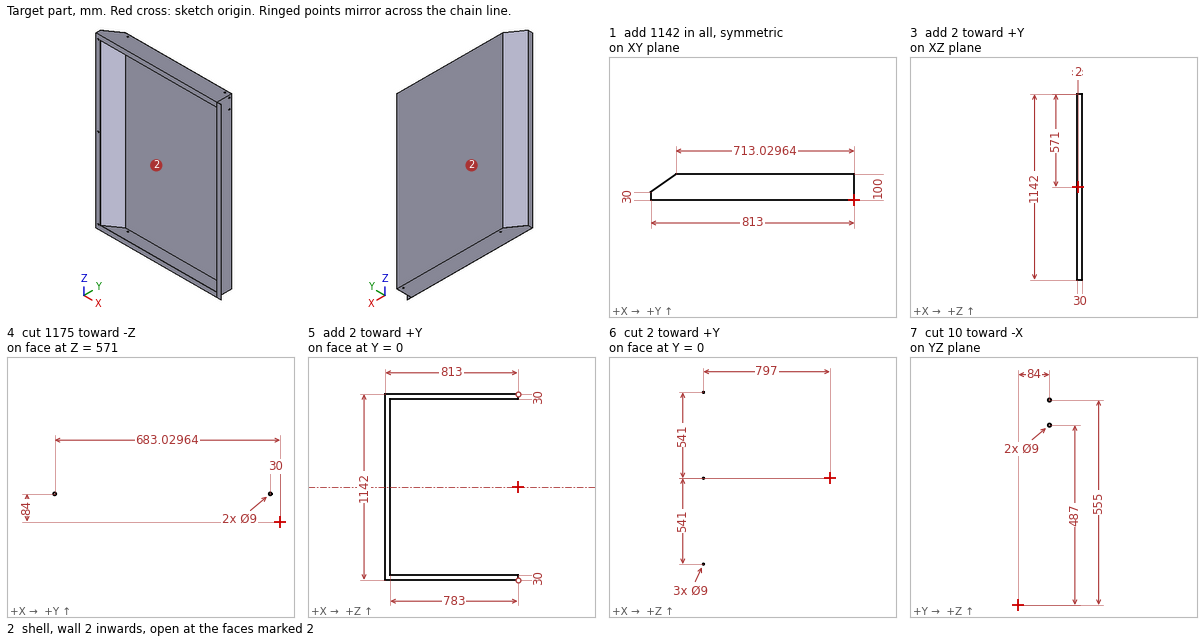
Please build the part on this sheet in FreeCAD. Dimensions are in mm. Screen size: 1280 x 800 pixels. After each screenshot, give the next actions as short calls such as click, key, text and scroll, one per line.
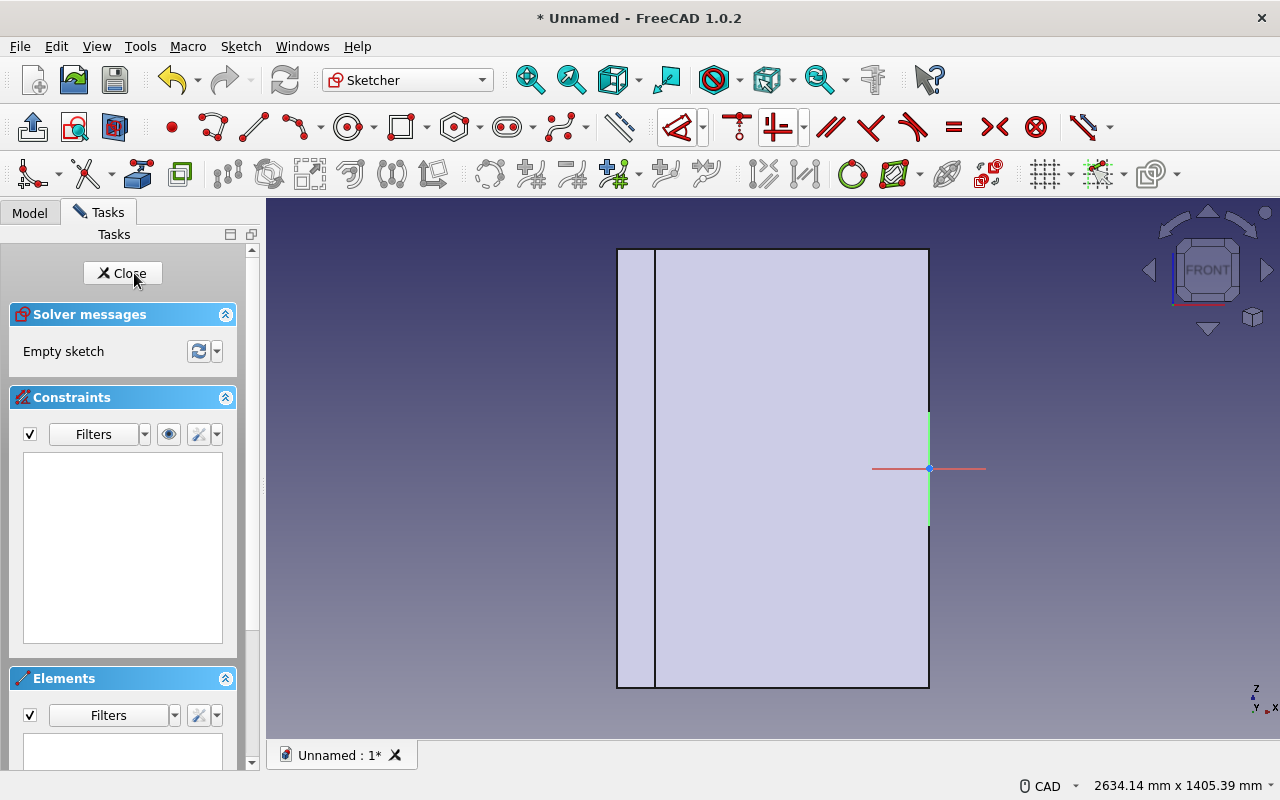
scroll(294, 468, down, 1)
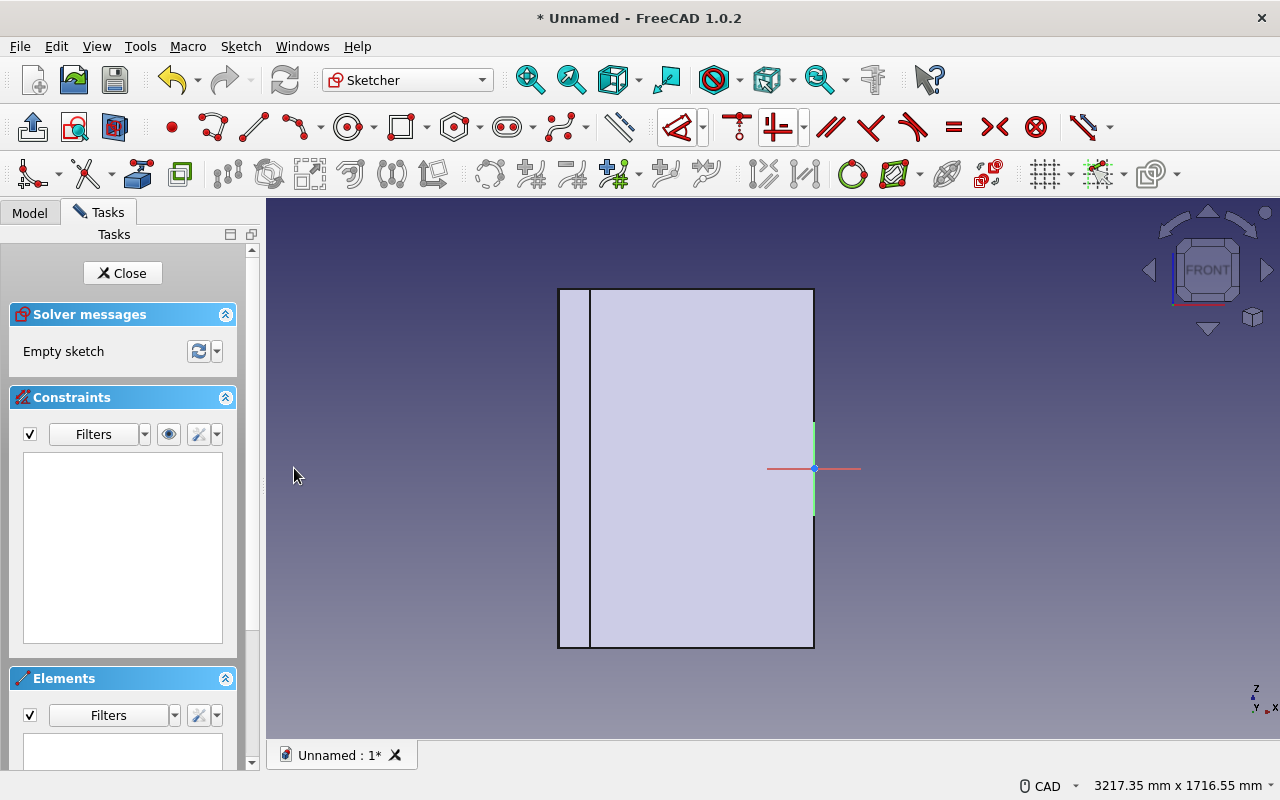
click(400, 128)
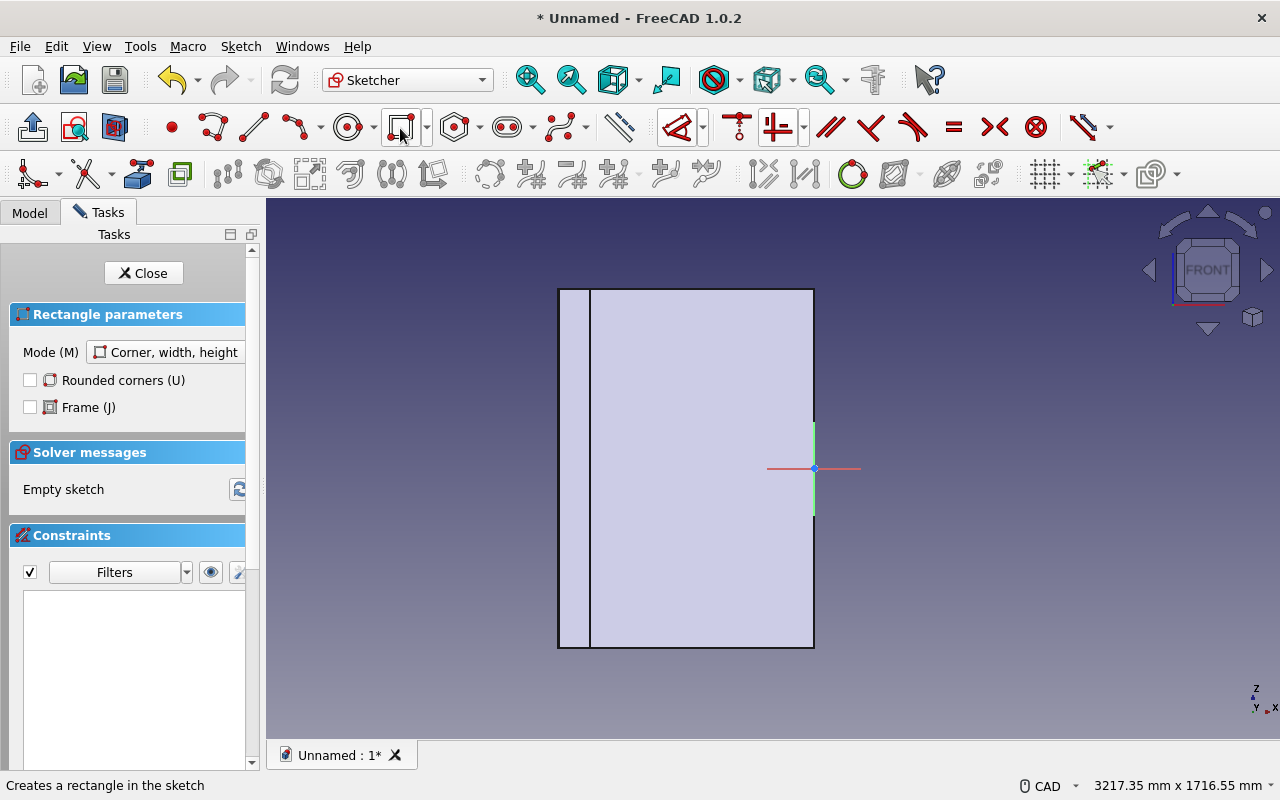
scroll(814, 289, up, 17)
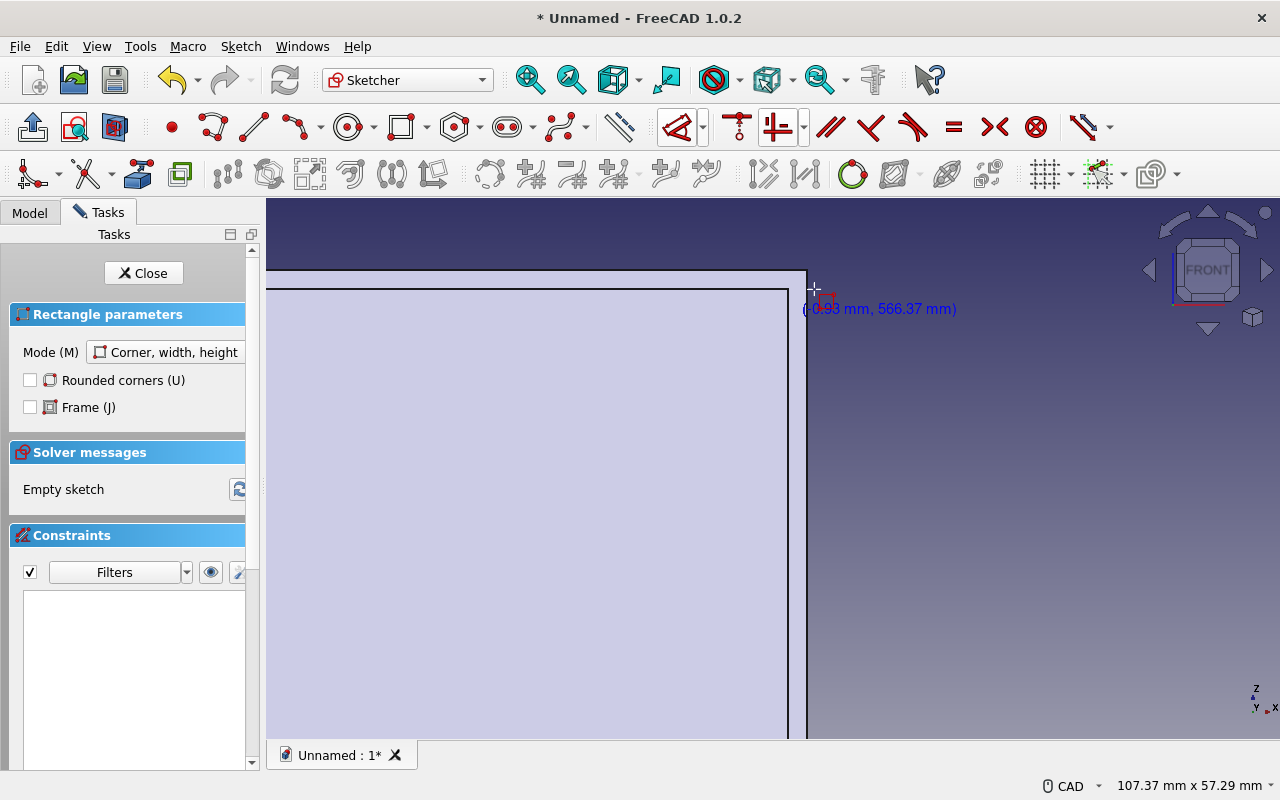
click(788, 270)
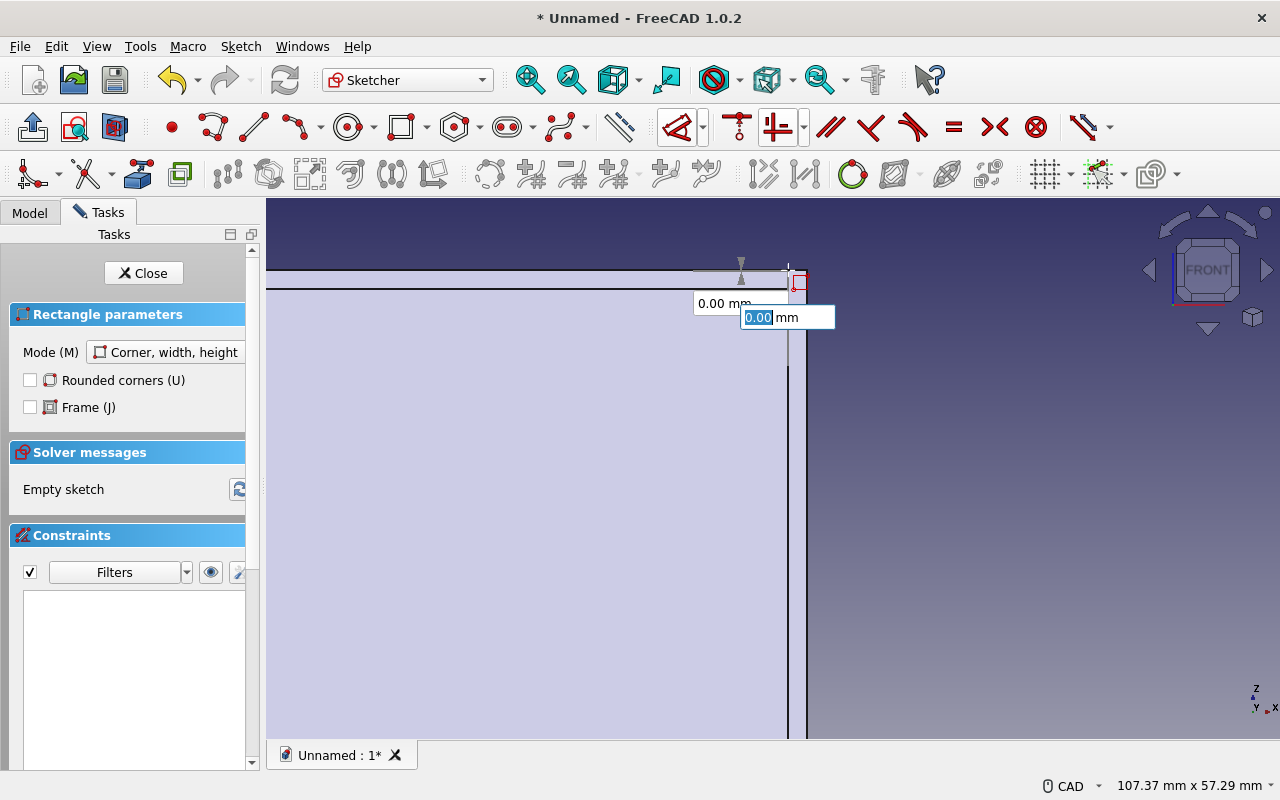
scroll(697, 289, down, 17)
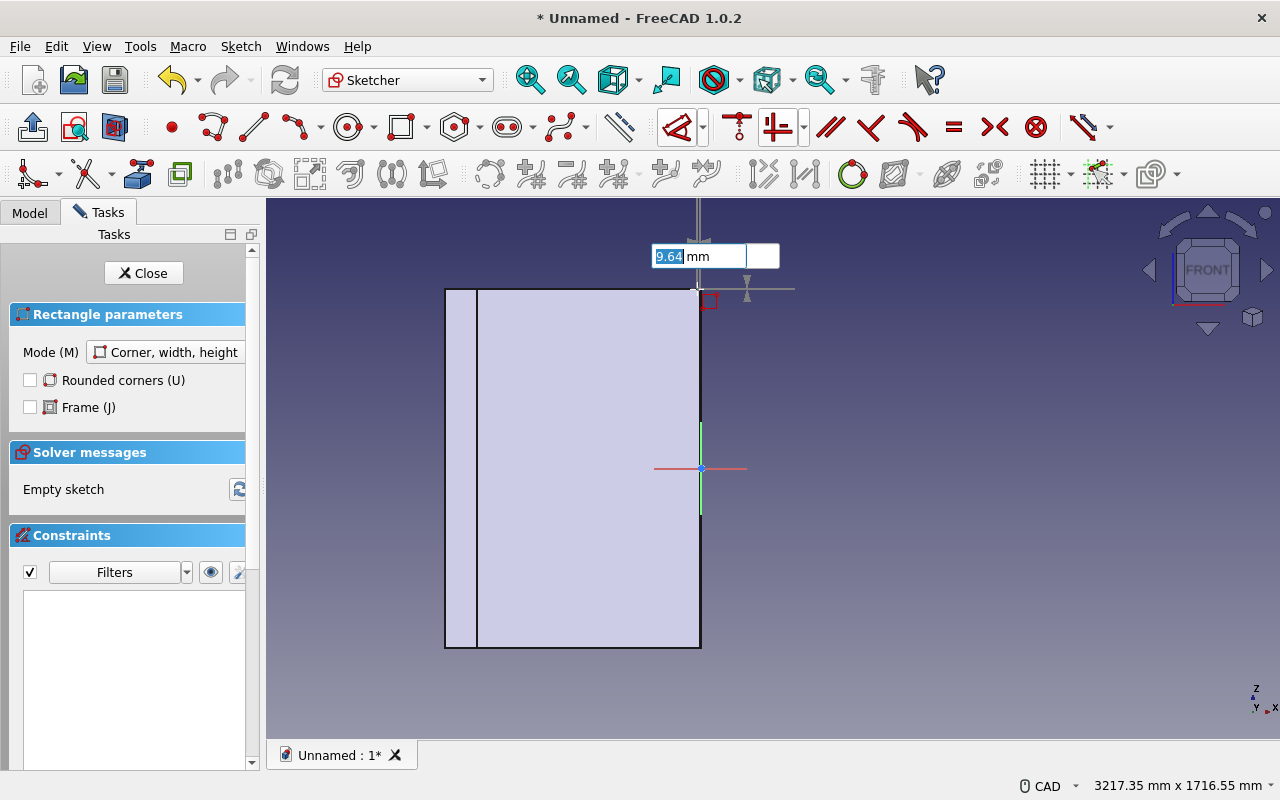
scroll(710, 648, up, 3)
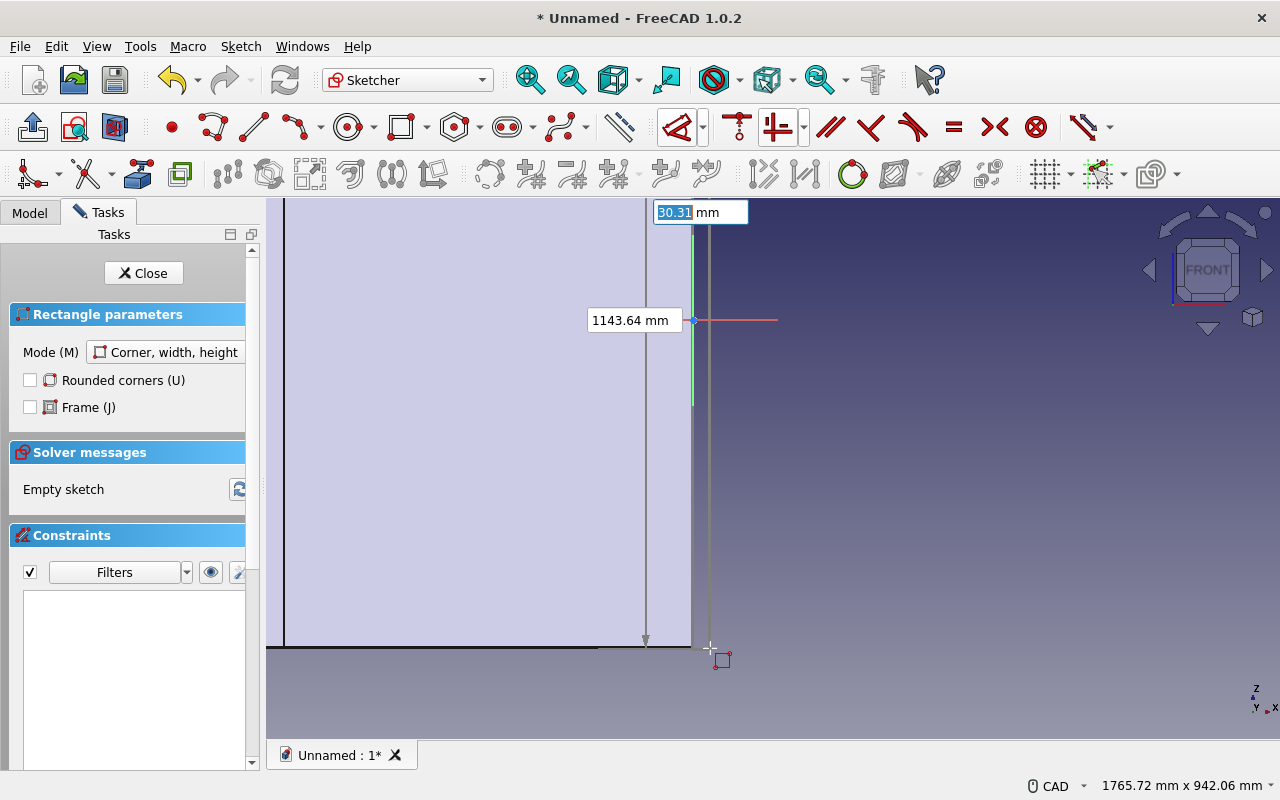
click(709, 648)
key(Escape)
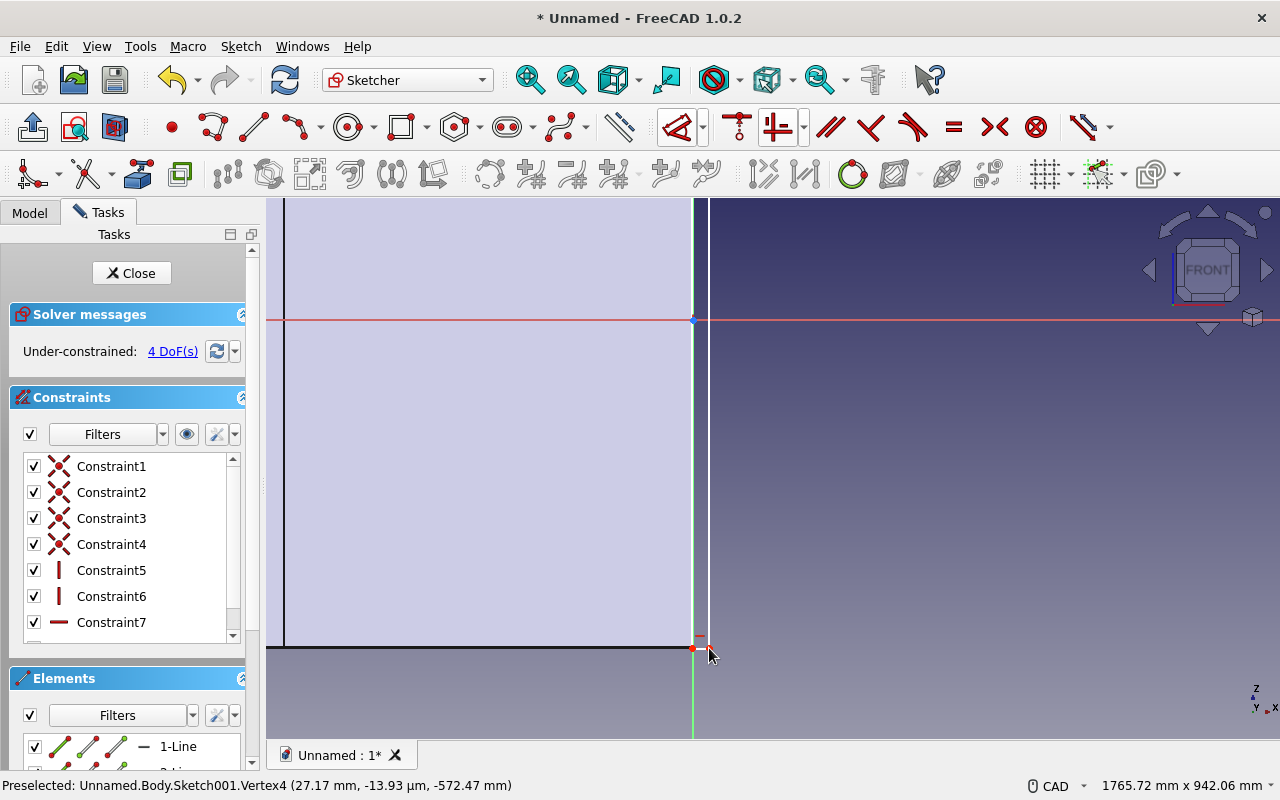
scroll(701, 649, up, 5)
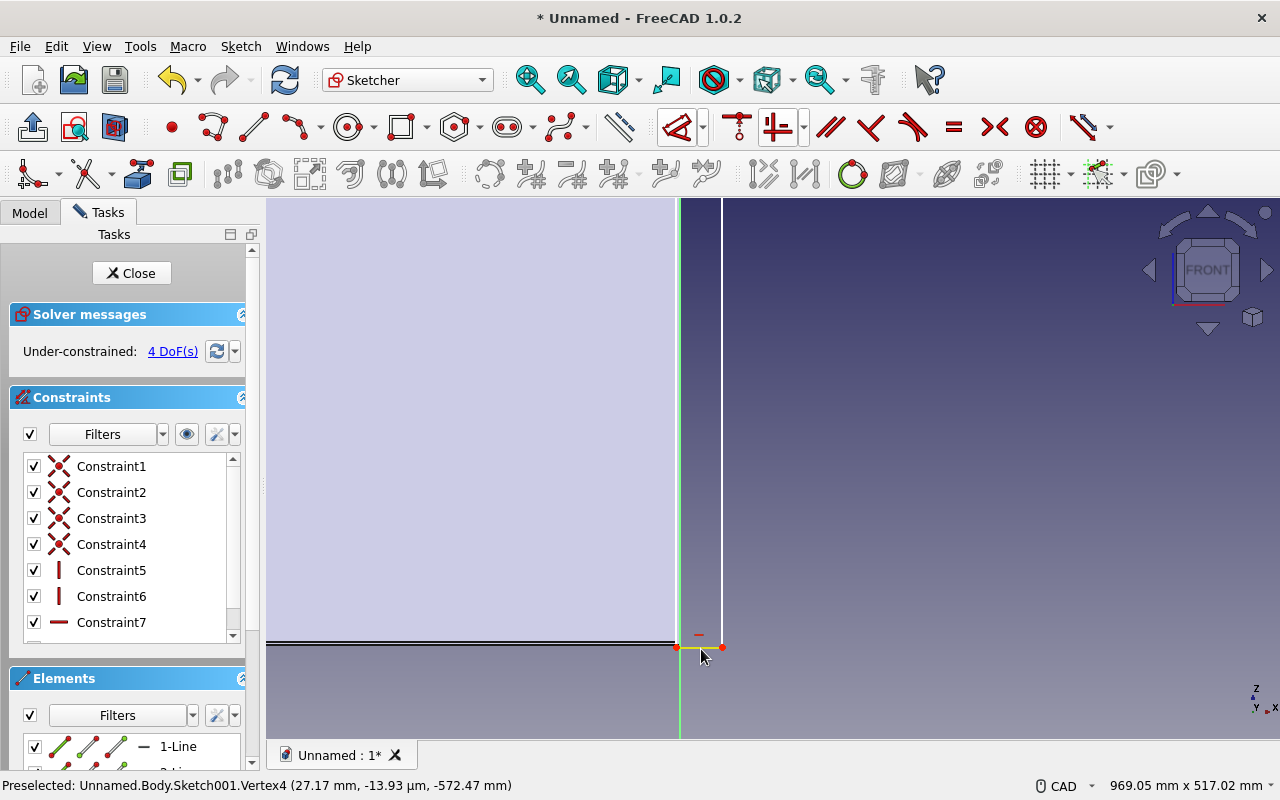
click(699, 648)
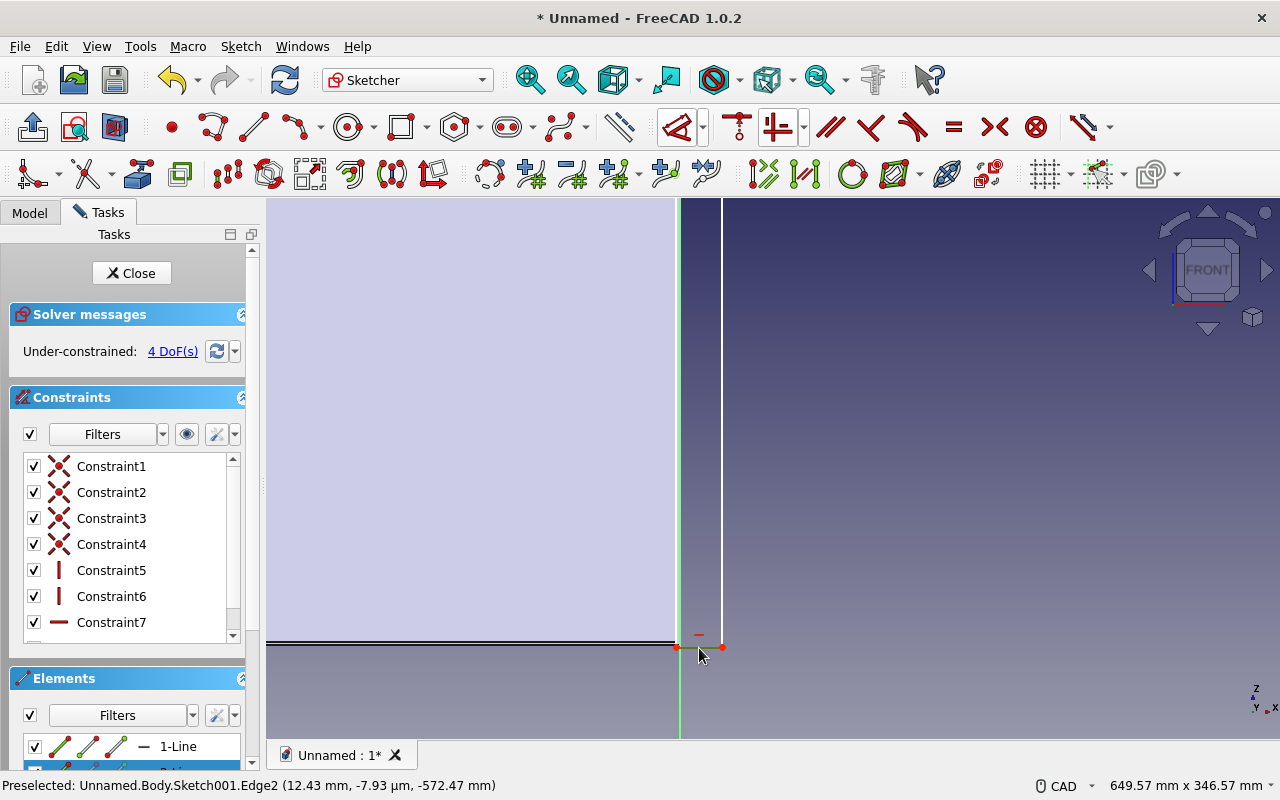
click(702, 128)